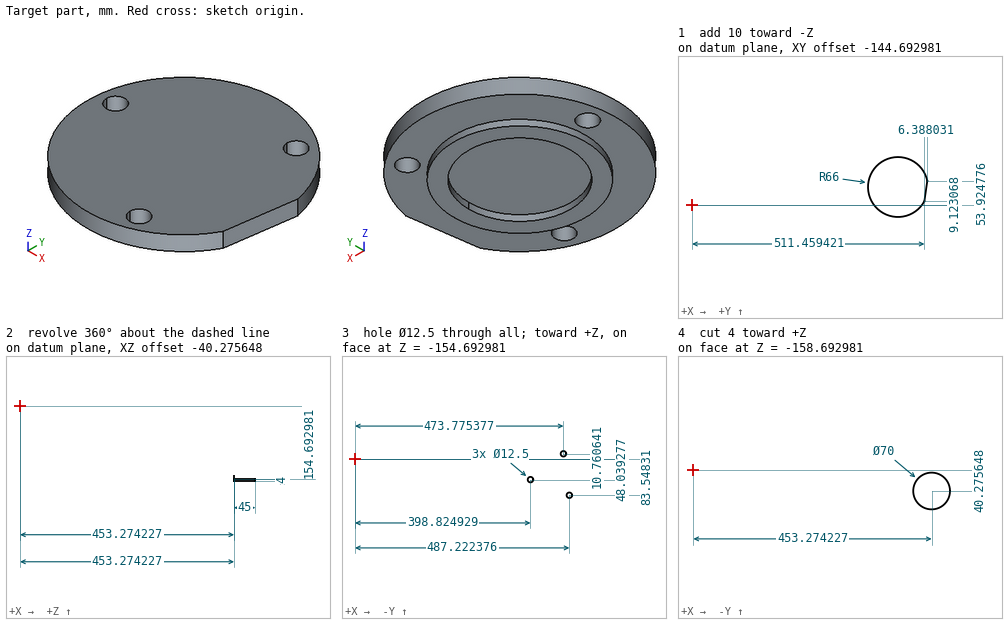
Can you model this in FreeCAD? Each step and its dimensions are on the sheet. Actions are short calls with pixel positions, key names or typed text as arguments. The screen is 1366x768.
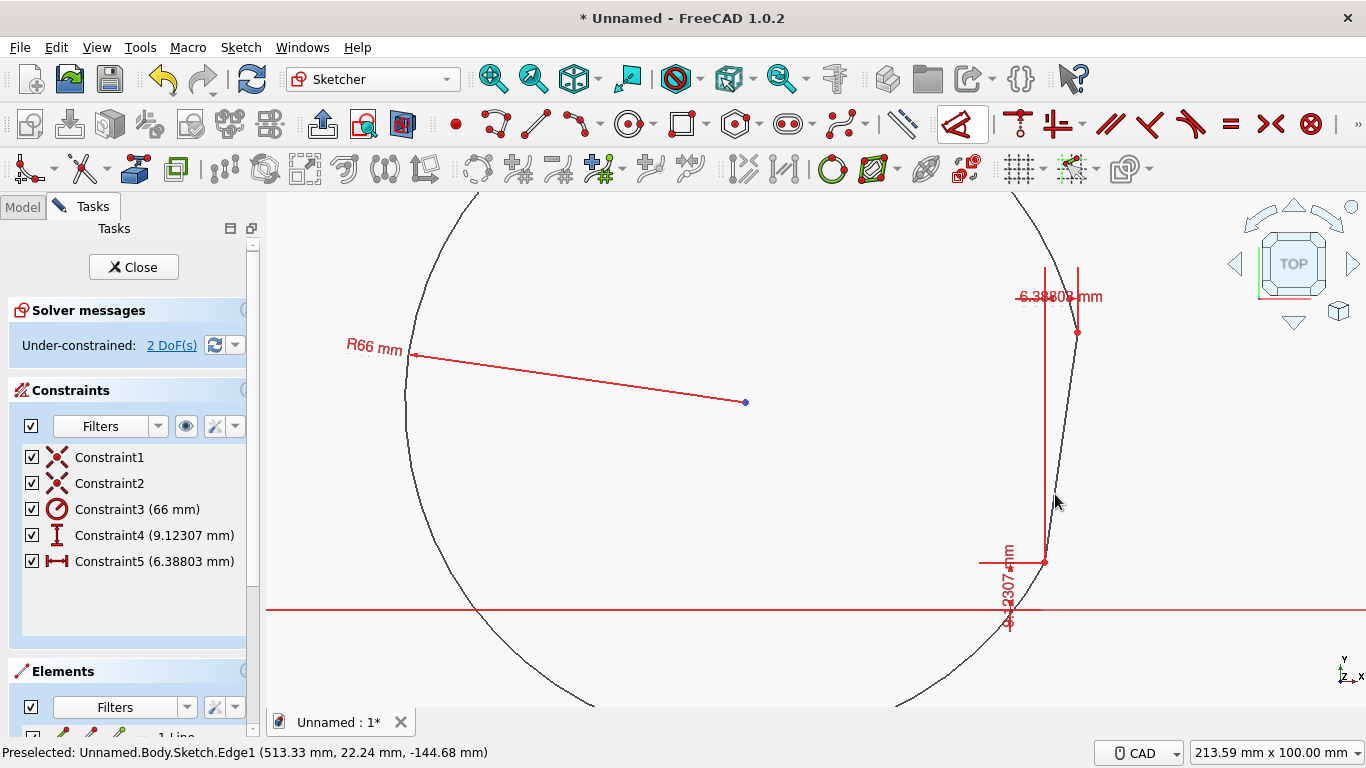
click(1078, 333)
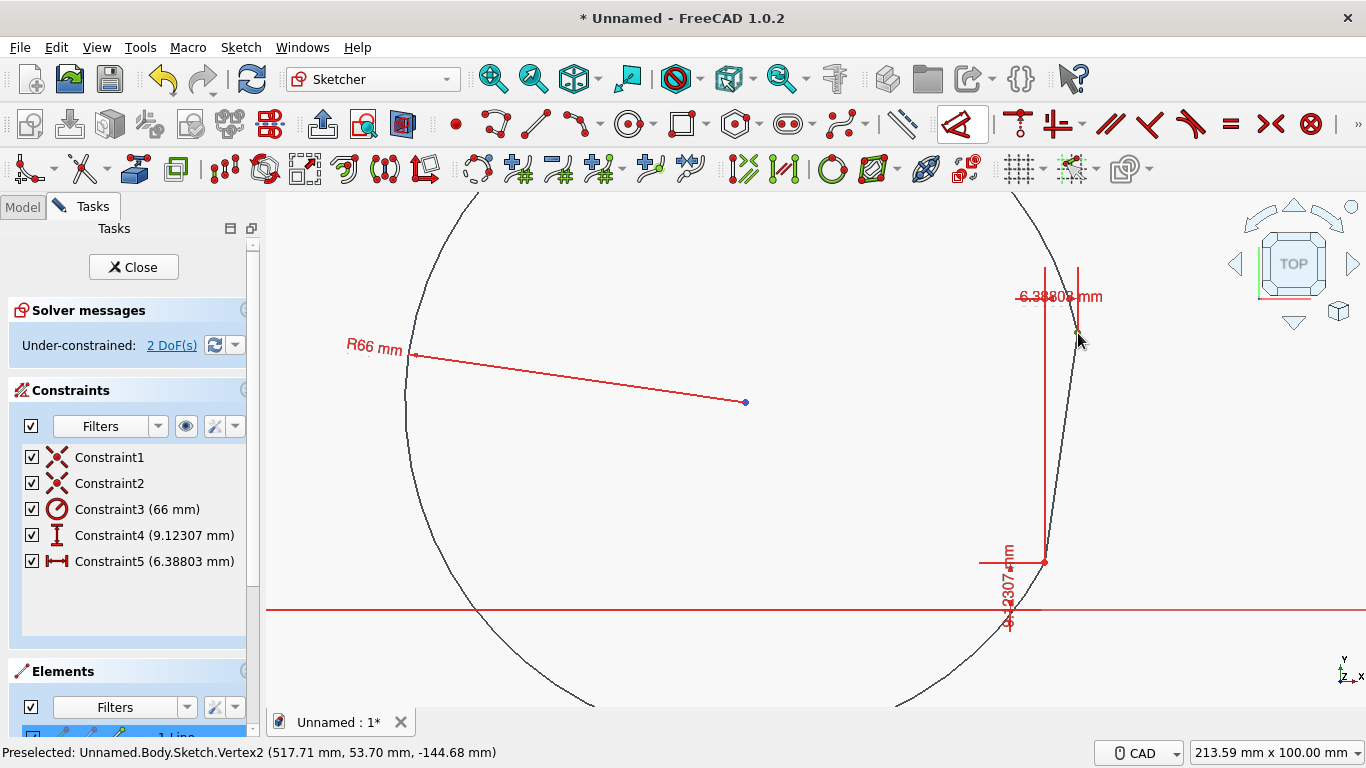
key(i)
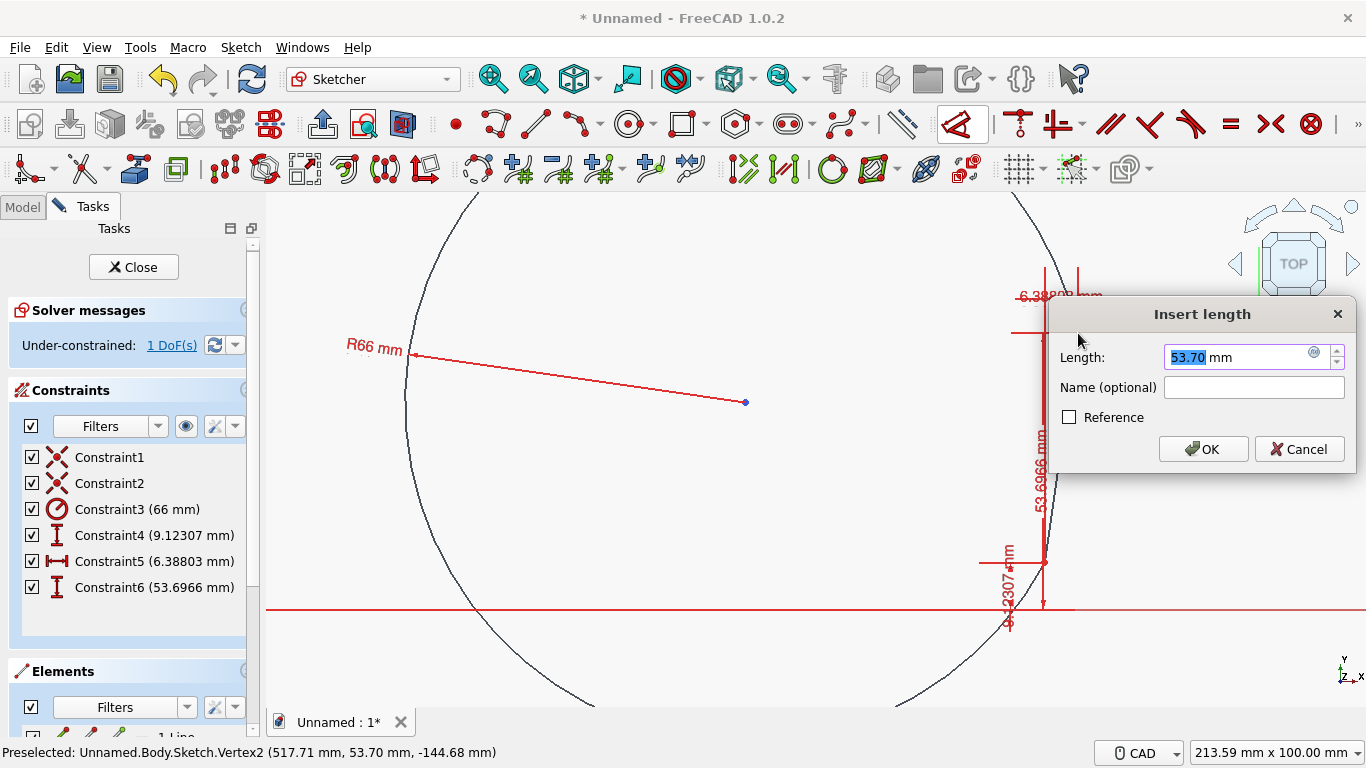
text(53.924776)
key(Return)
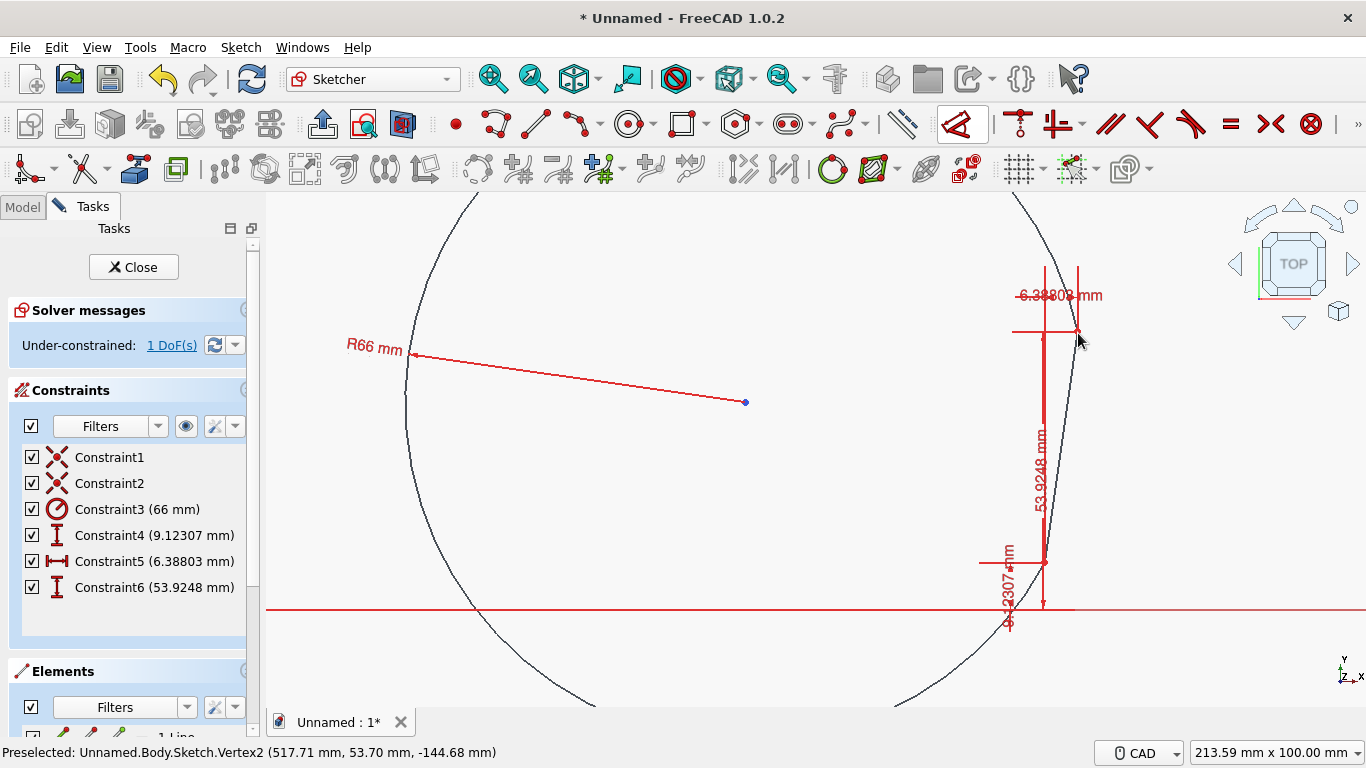
click(1045, 563)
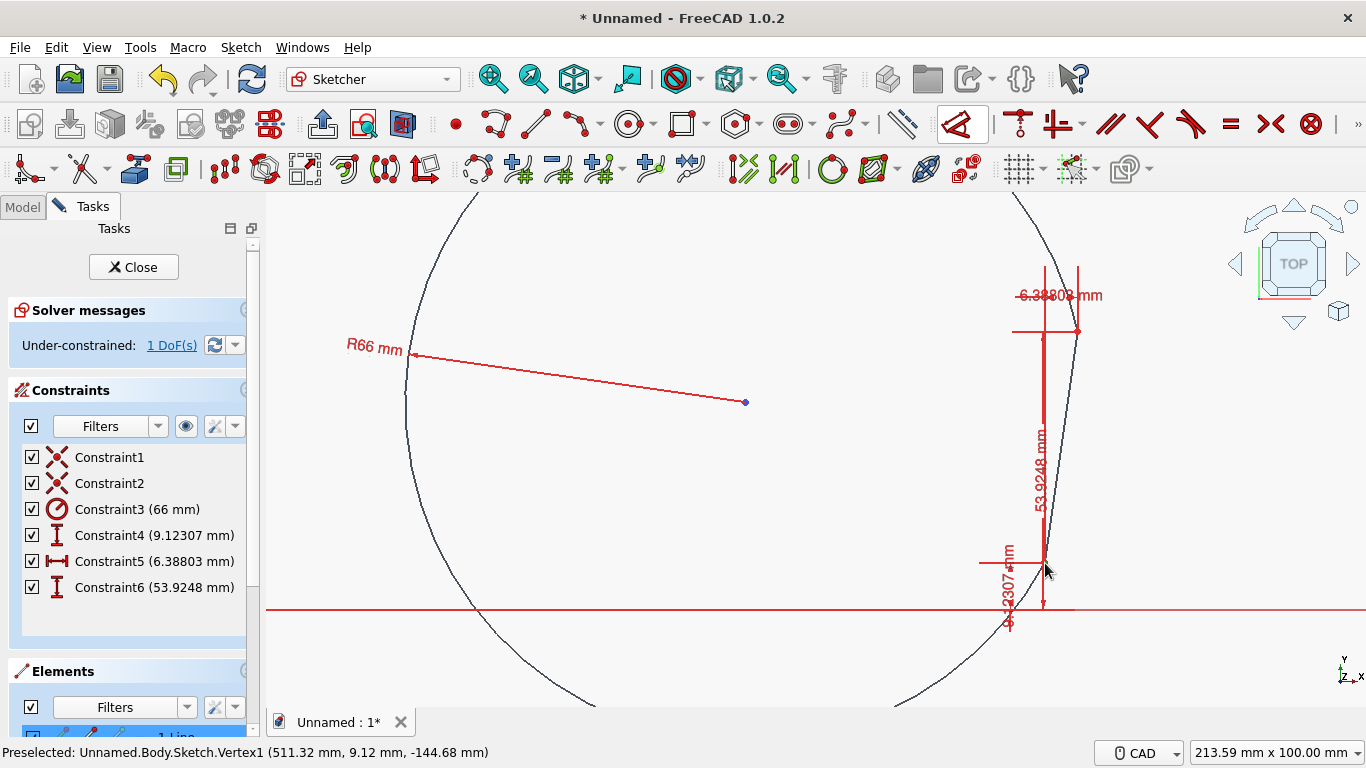
click(982, 124)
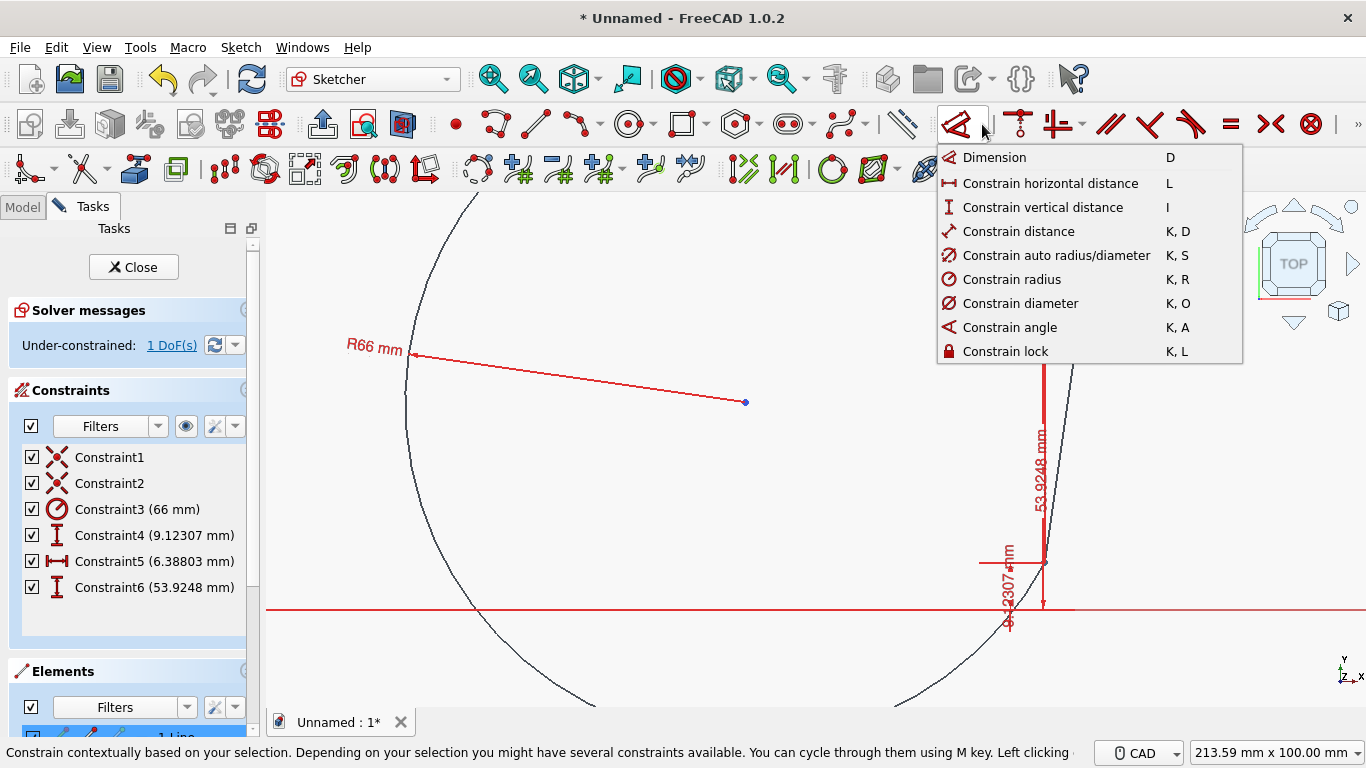
click(1090, 183)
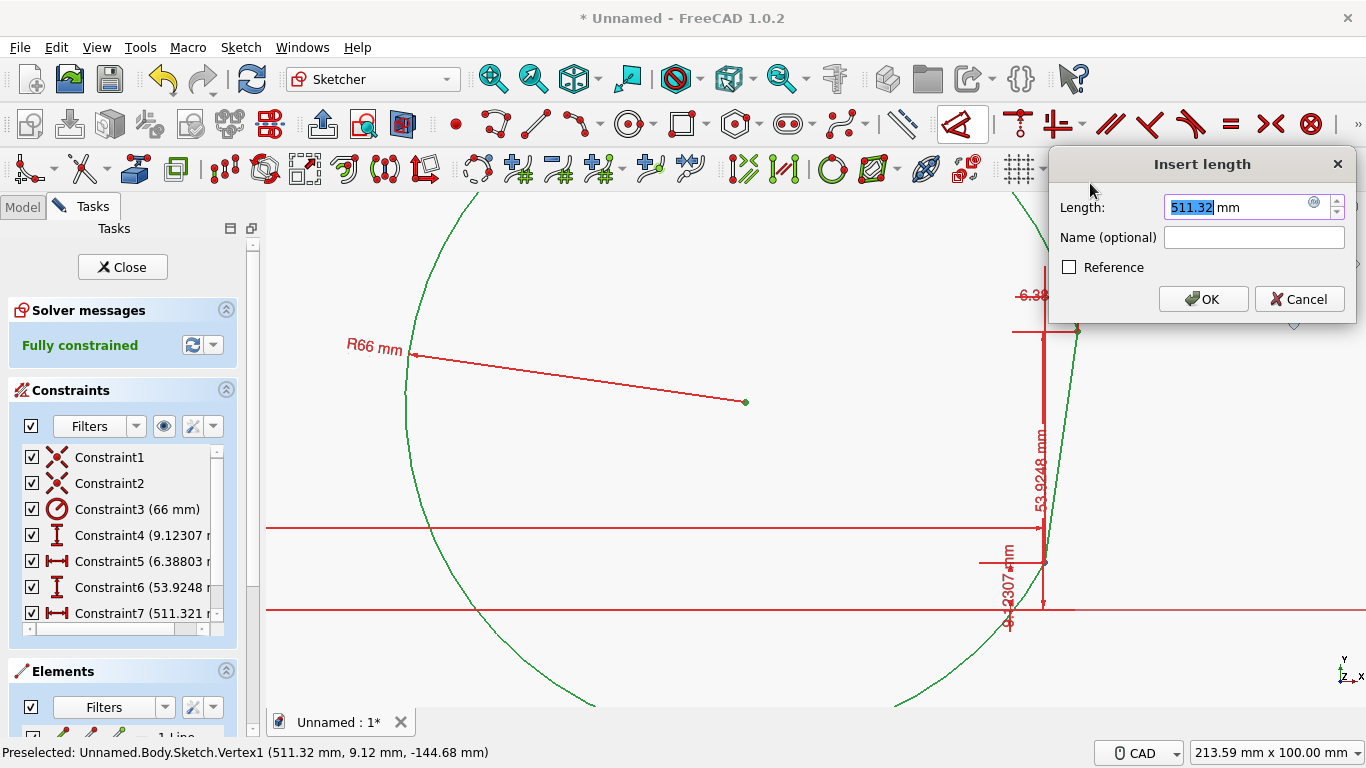
text(511.459421)
key(Return)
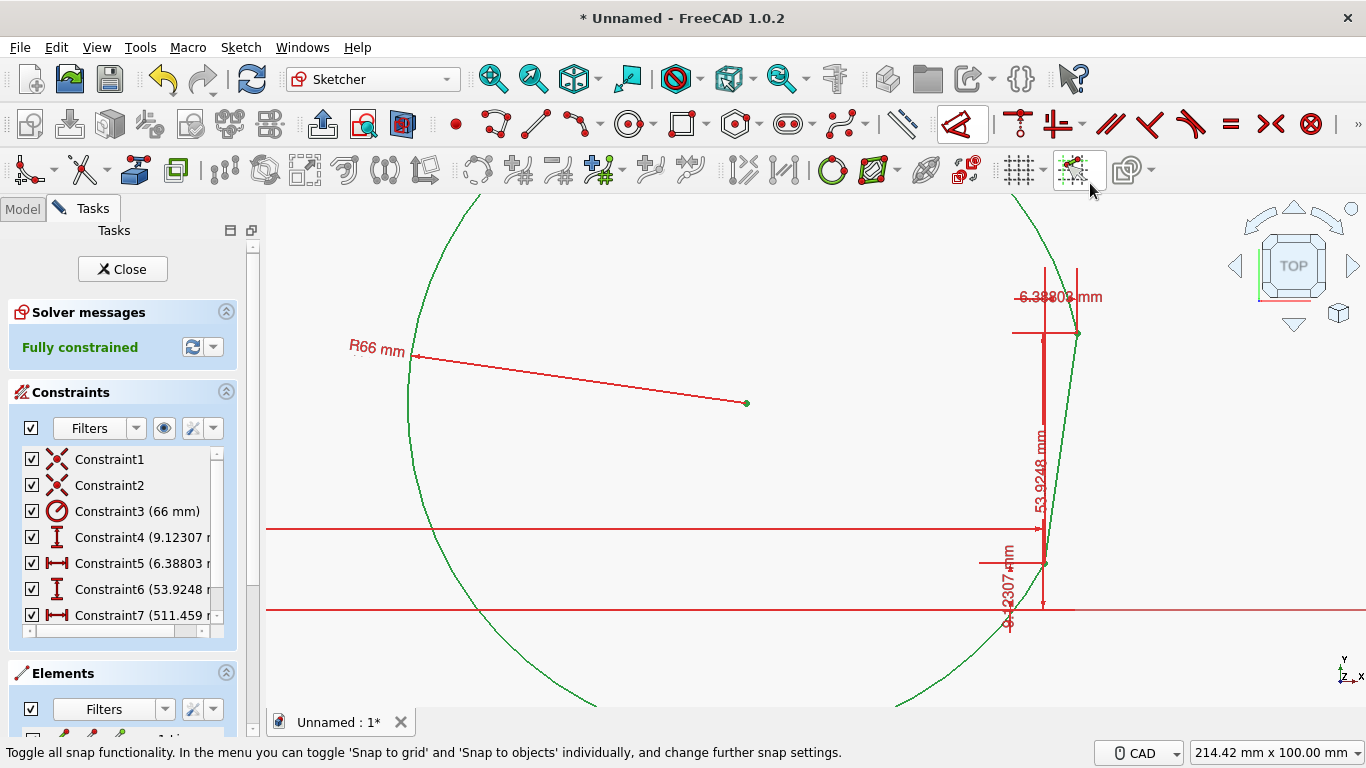
click(123, 269)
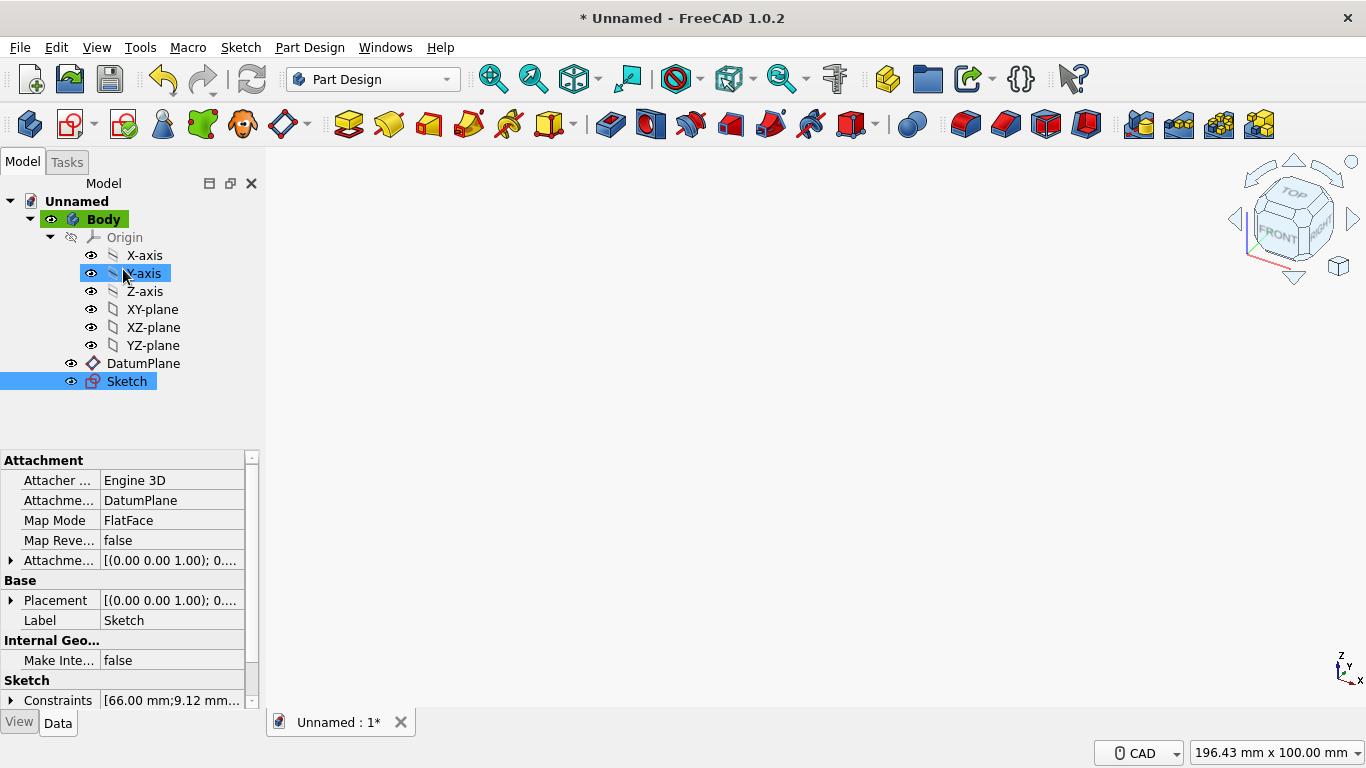
click(350, 124)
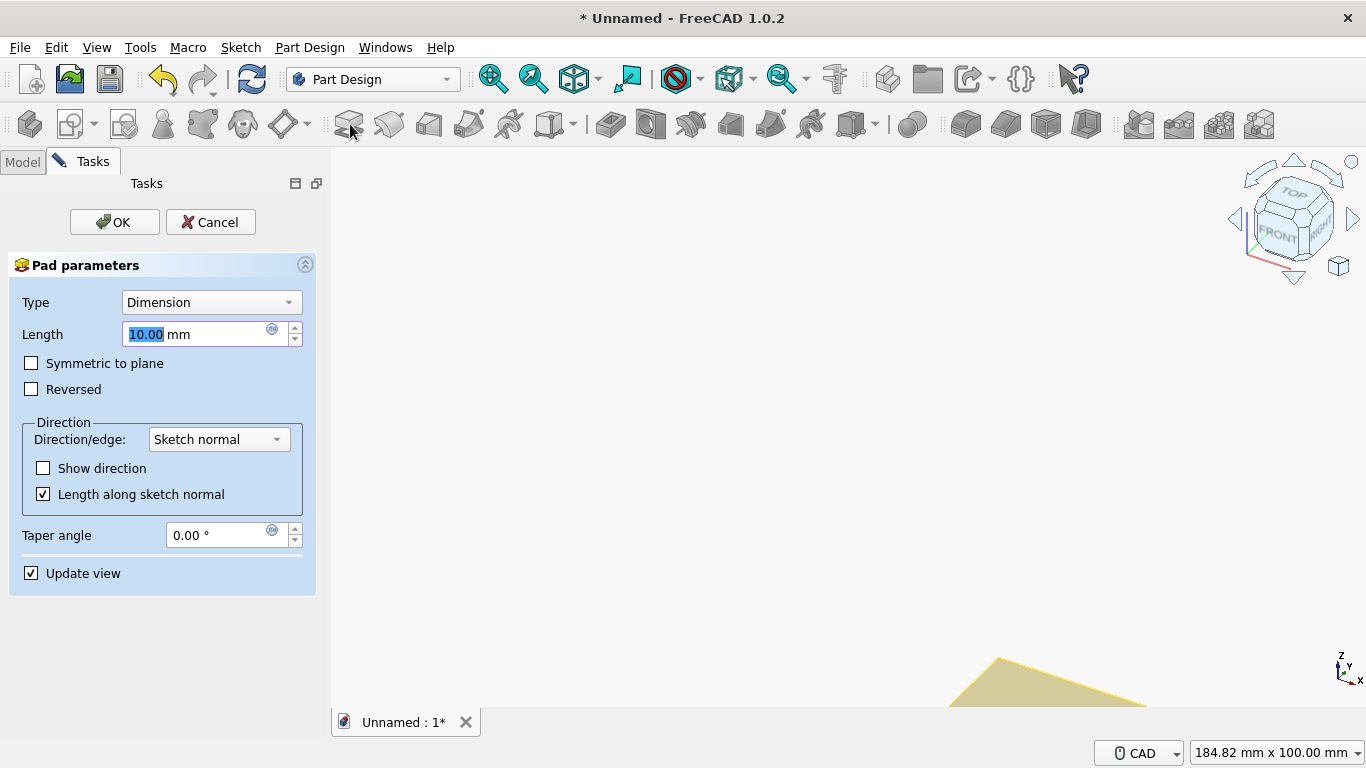
text(10)
key(Tab)